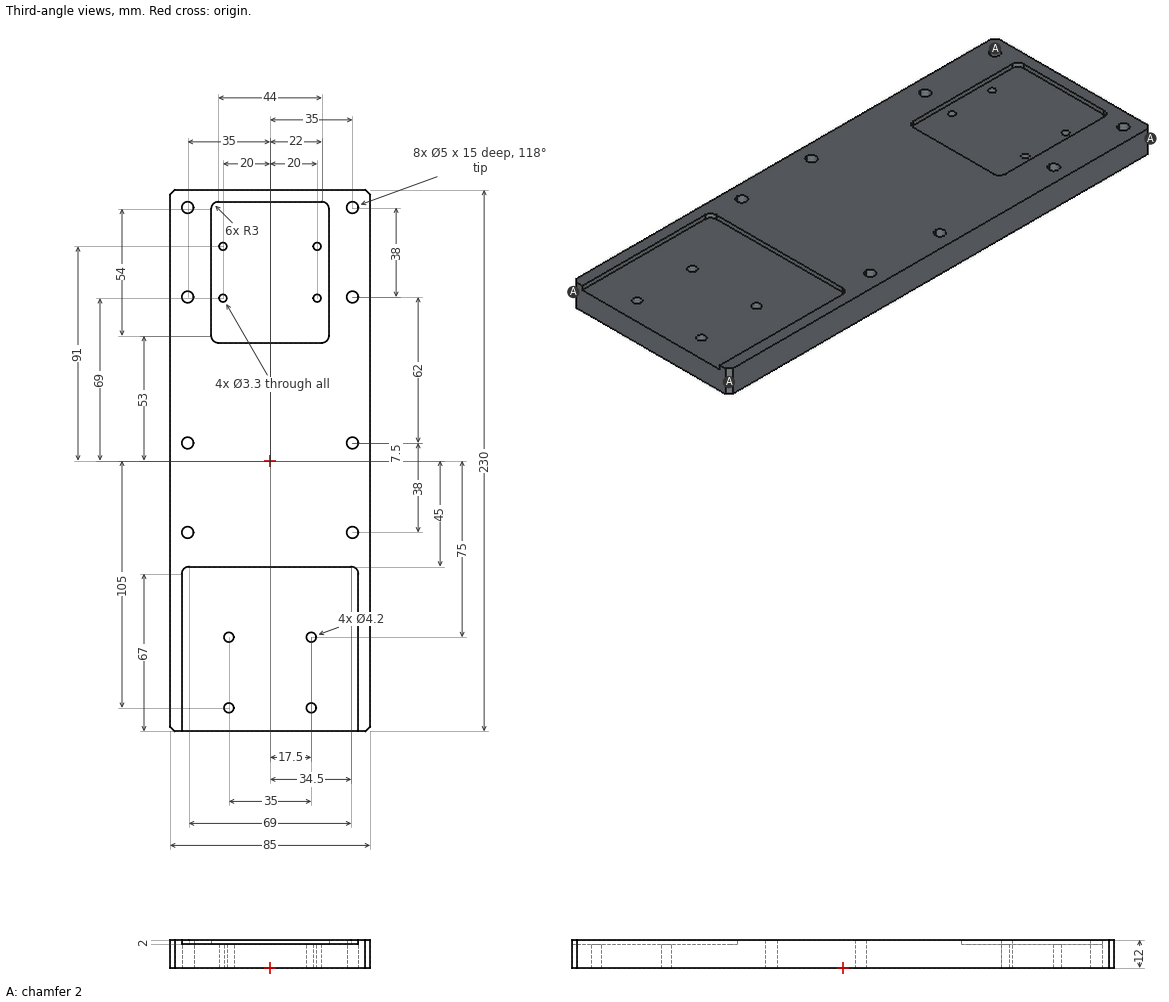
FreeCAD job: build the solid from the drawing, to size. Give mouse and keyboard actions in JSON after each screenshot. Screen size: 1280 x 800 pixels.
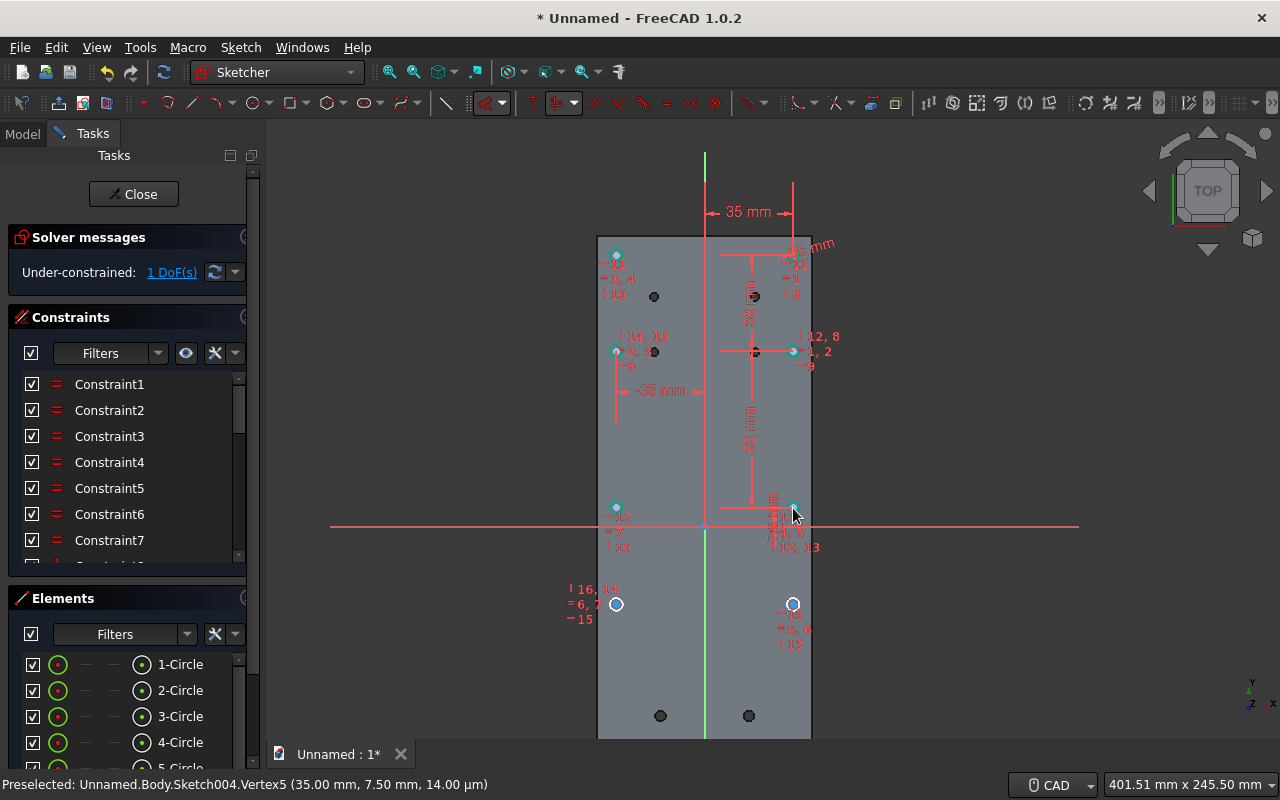
{"action": "left_click", "coordinate": [793, 508]}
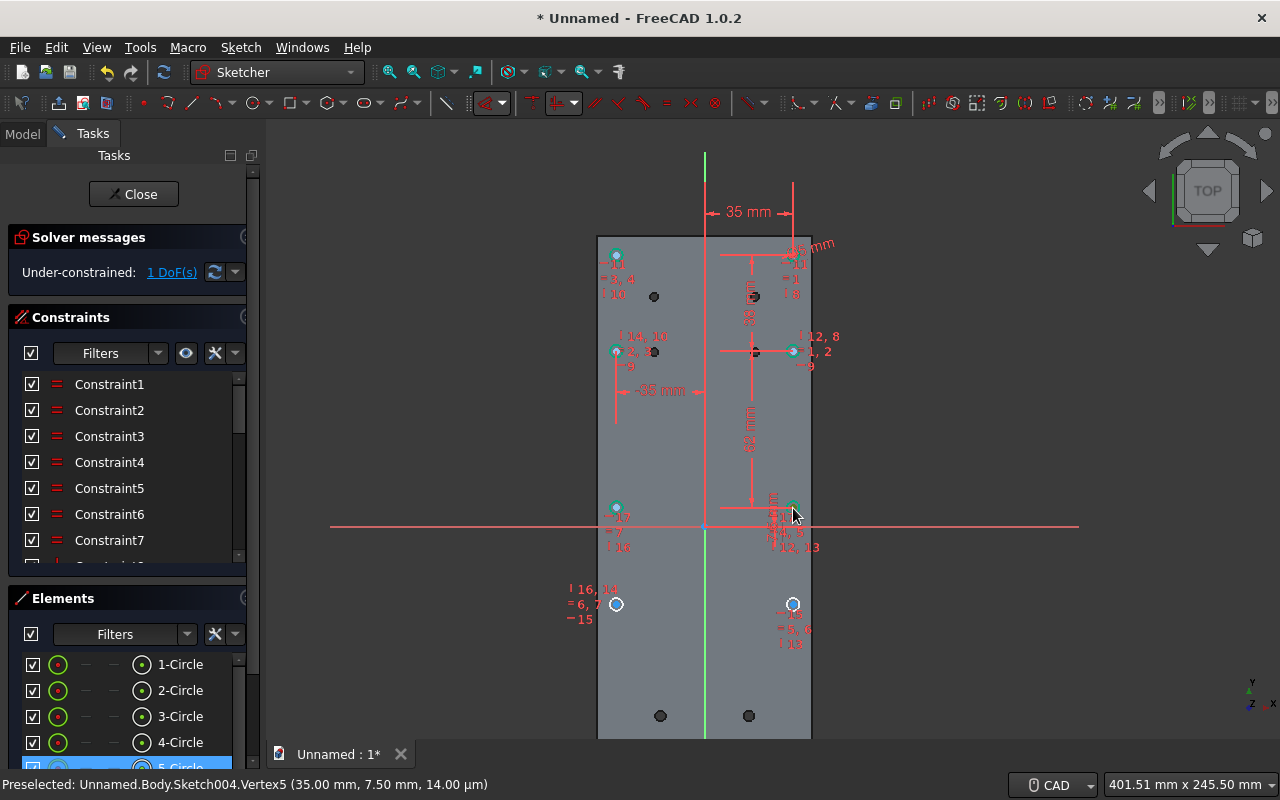
{"action": "left_click", "coordinate": [793, 604]}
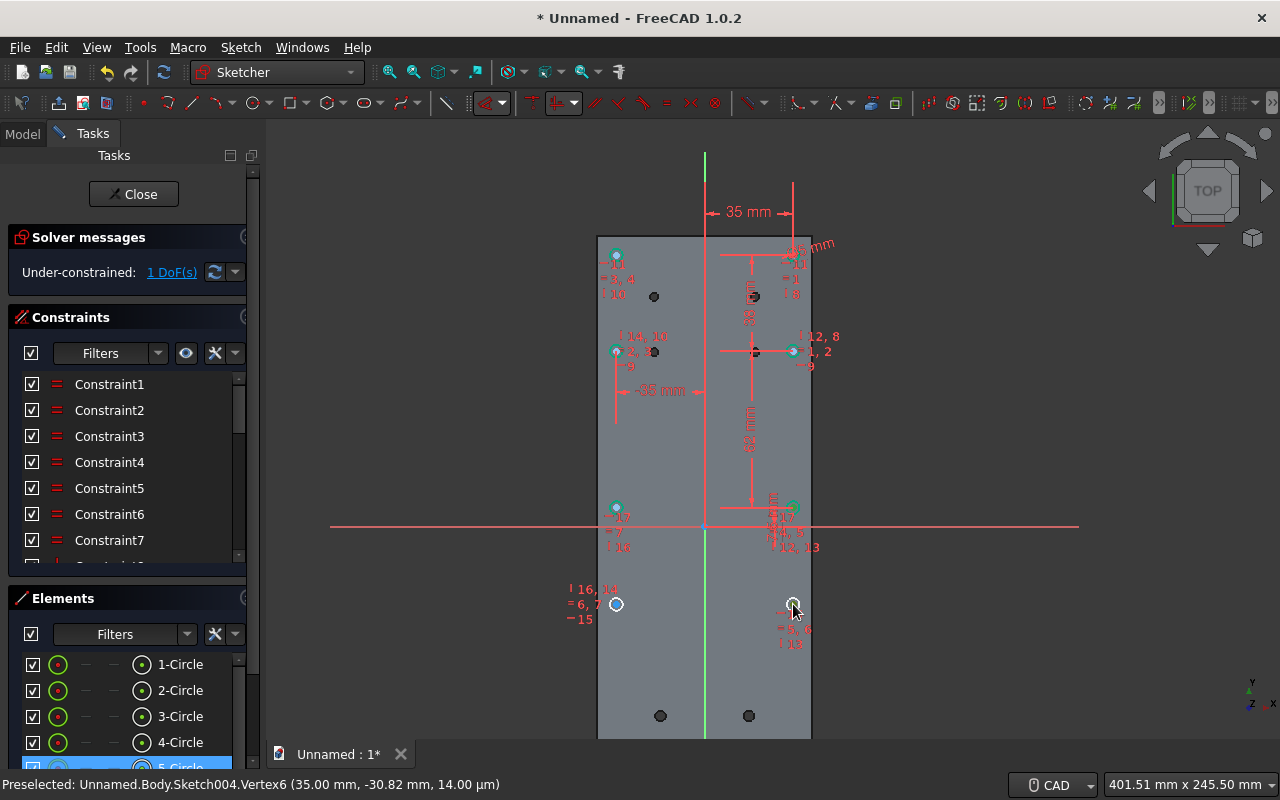
{"action": "key", "text": "i"}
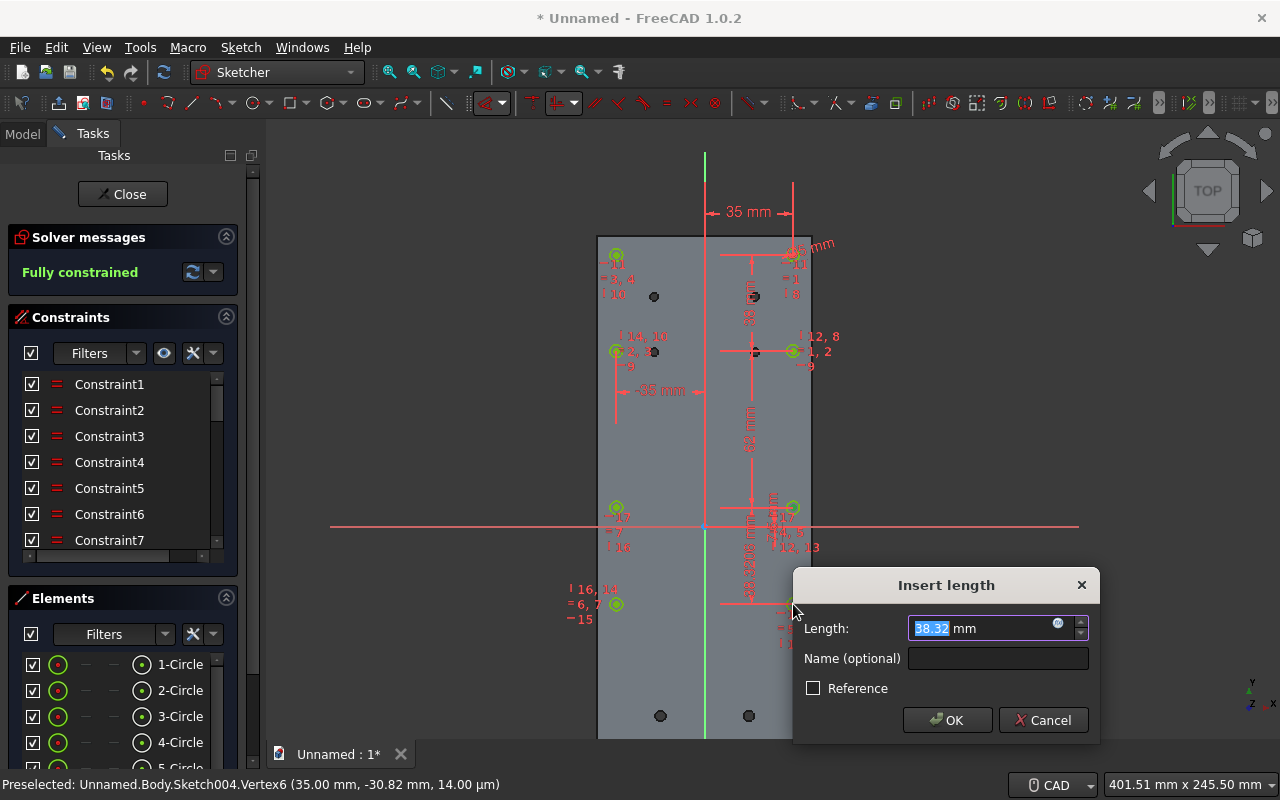
{"action": "type", "text": "38"}
{"action": "key", "text": "Return"}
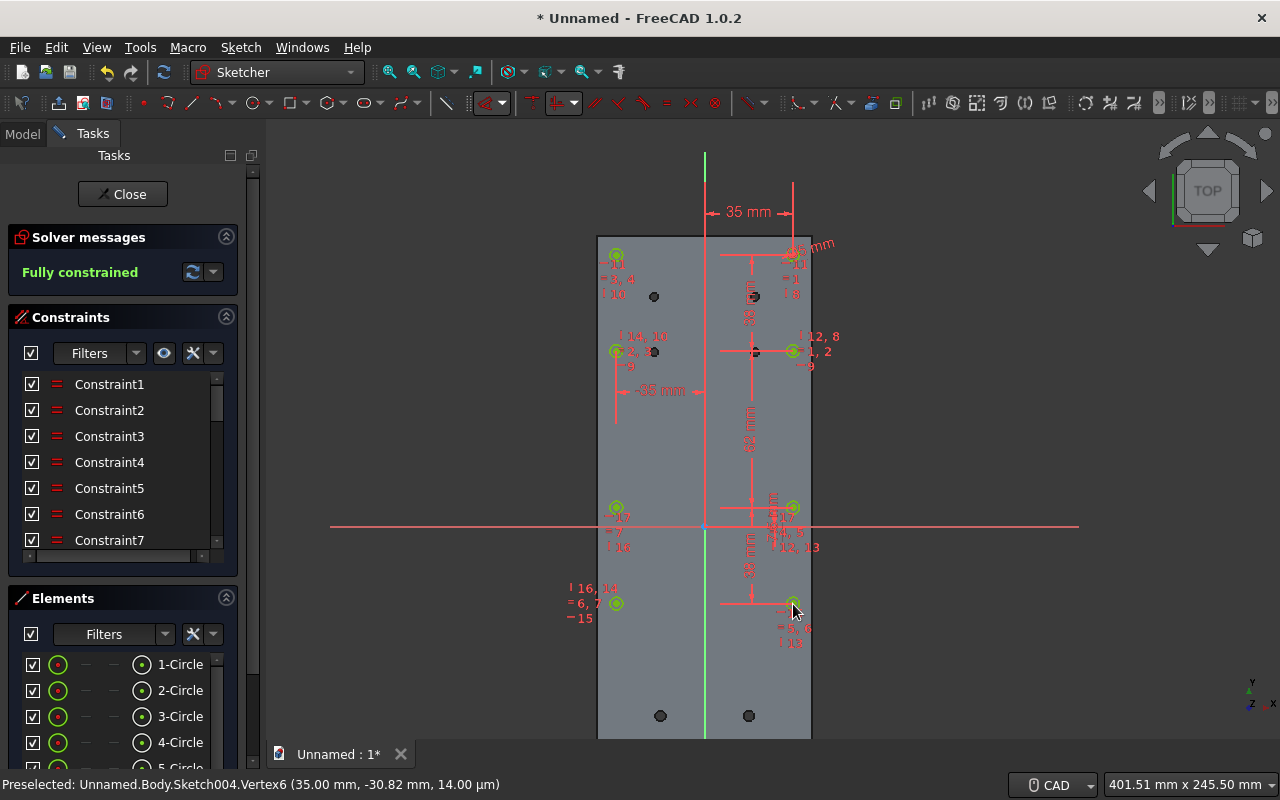
{"action": "left_click", "coordinate": [123, 194]}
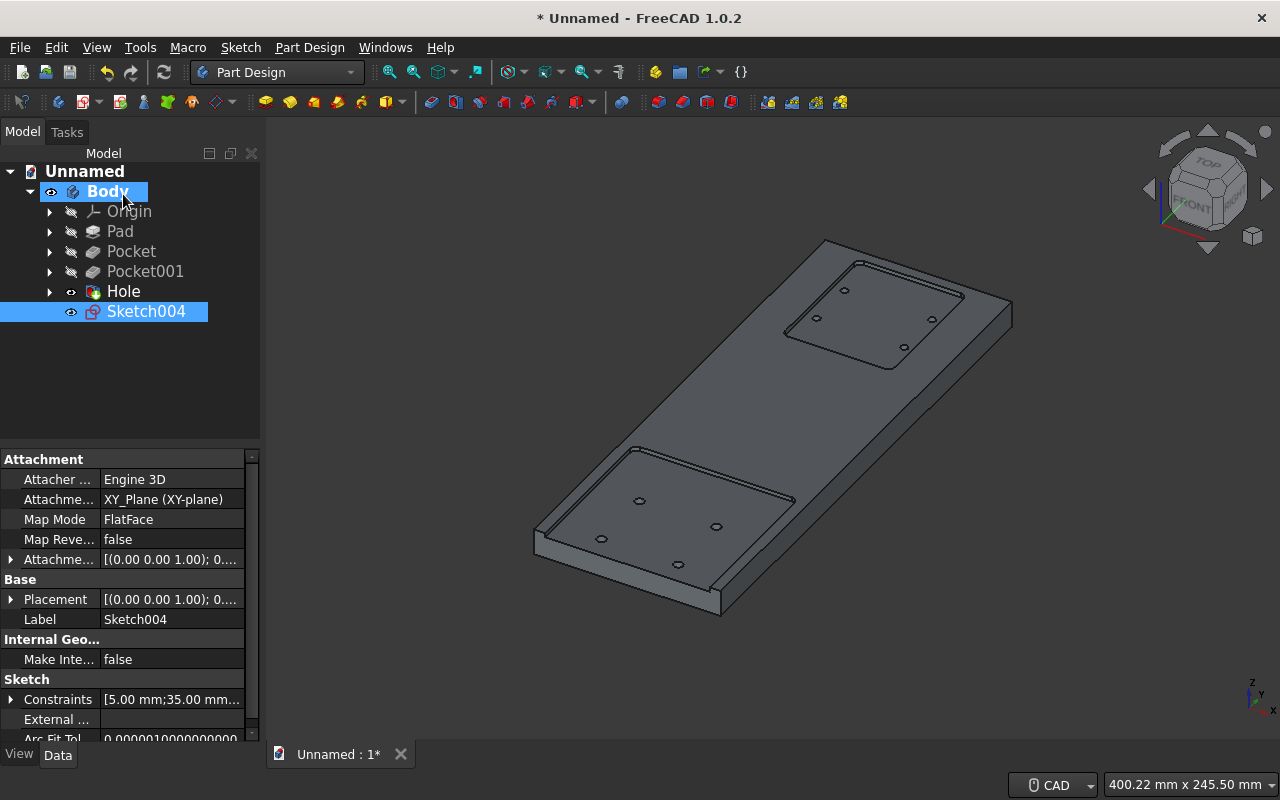
{"action": "left_click", "coordinate": [456, 102]}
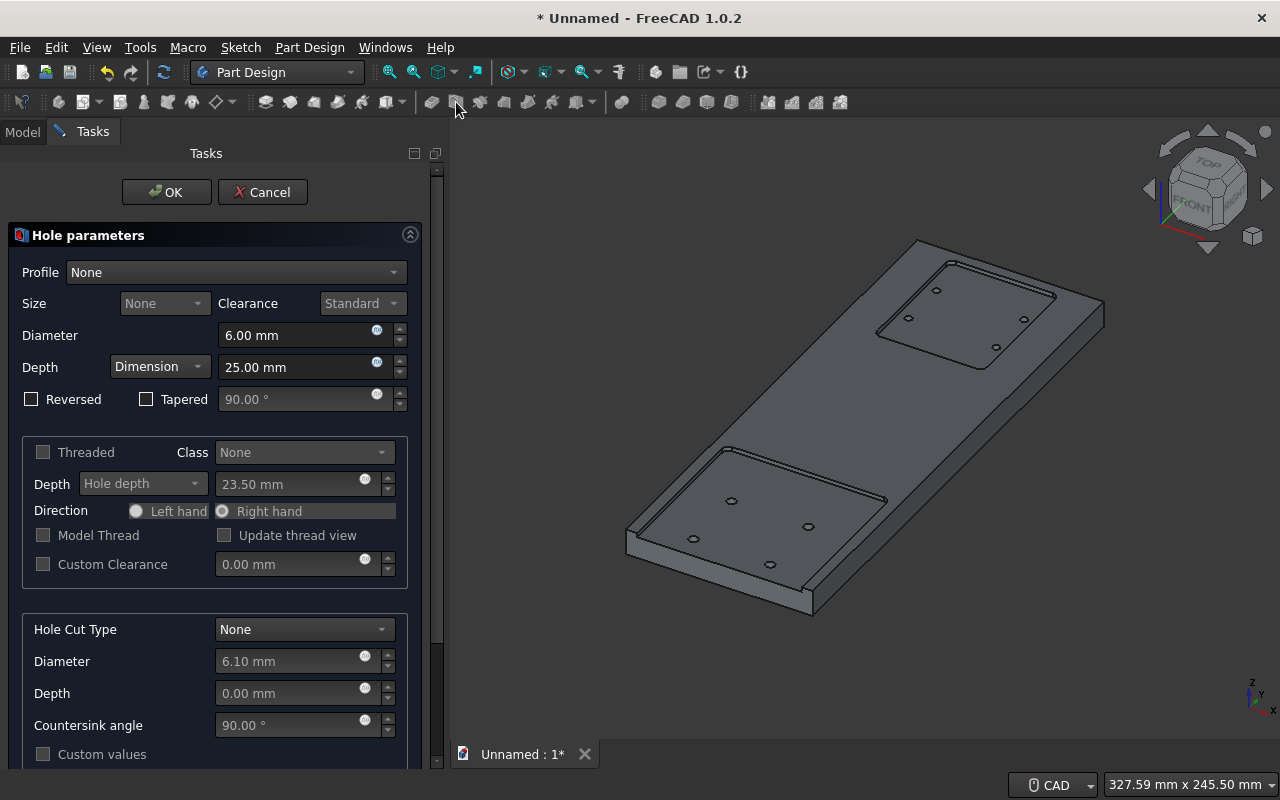
{"action": "triple_click", "coordinate": [305, 335]}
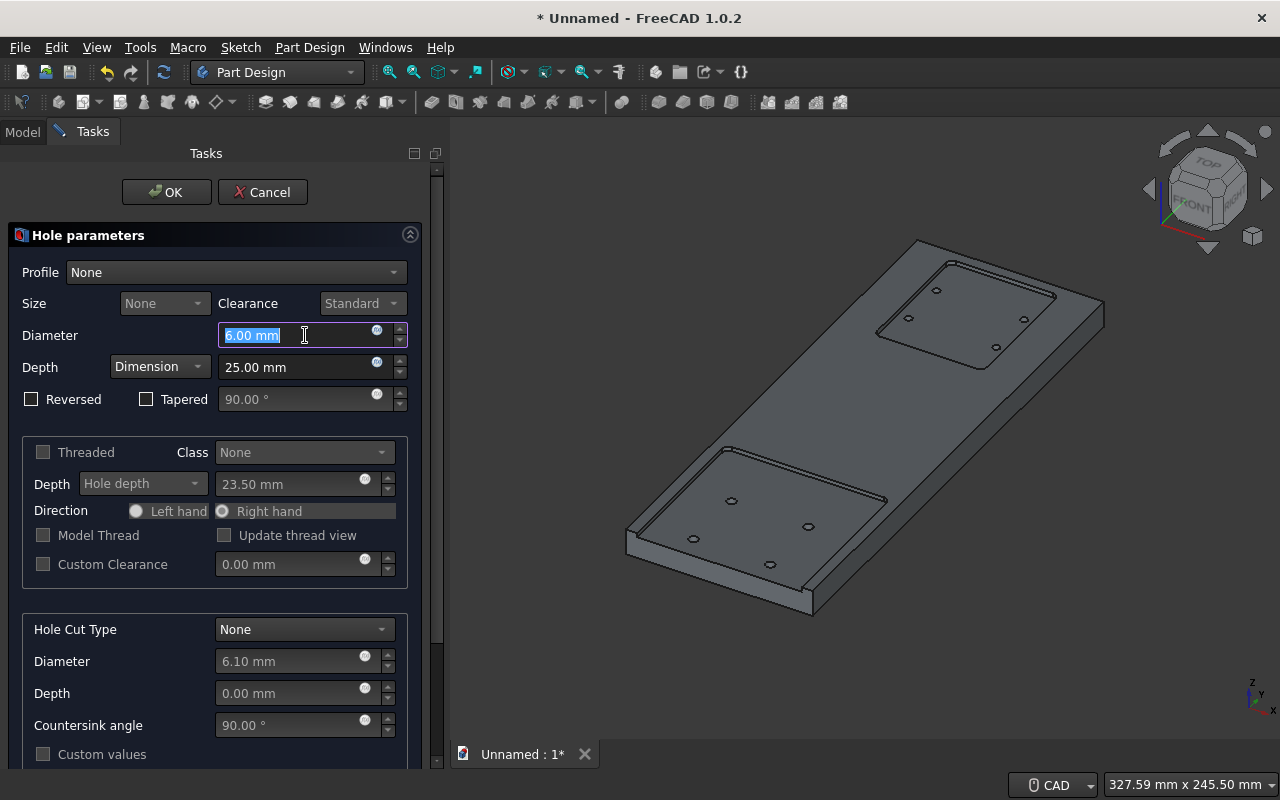
{"action": "type", "text": "5"}
{"action": "key", "text": "Tab"}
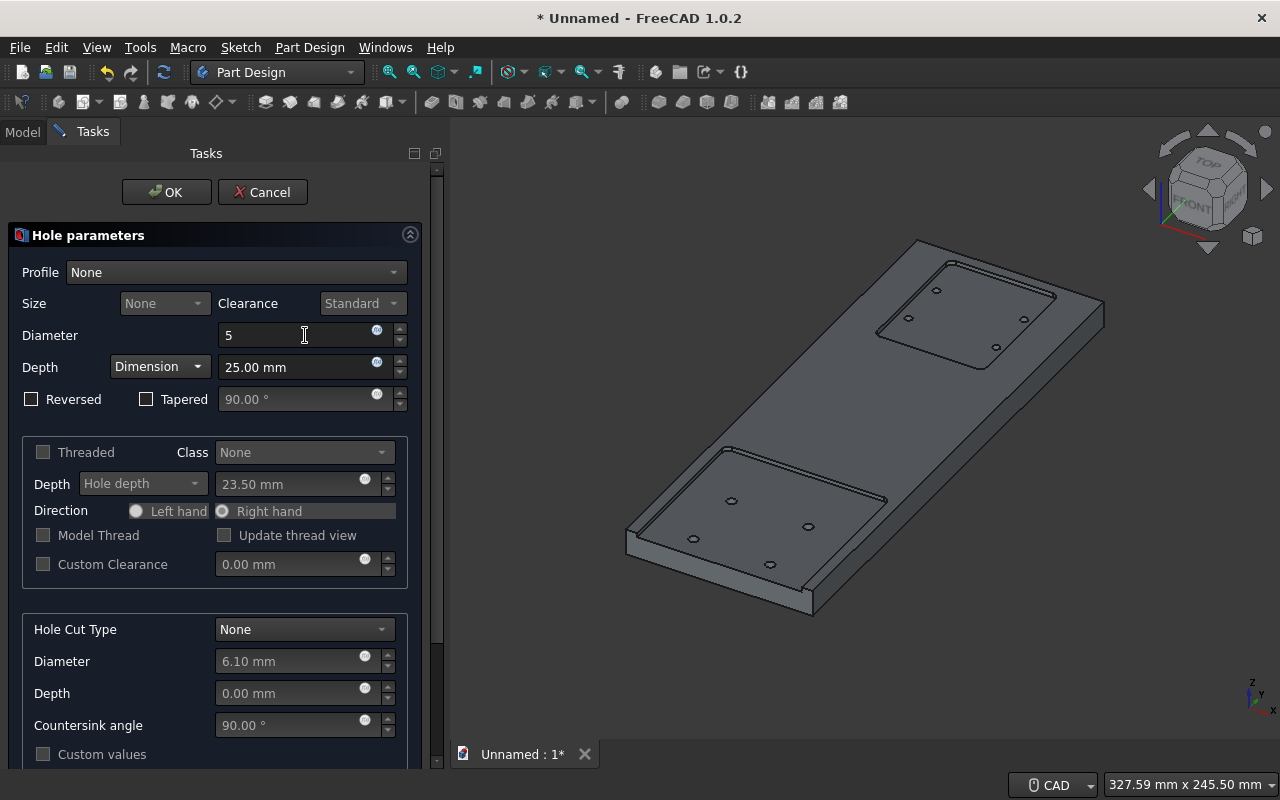
{"action": "triple_click", "coordinate": [305, 367]}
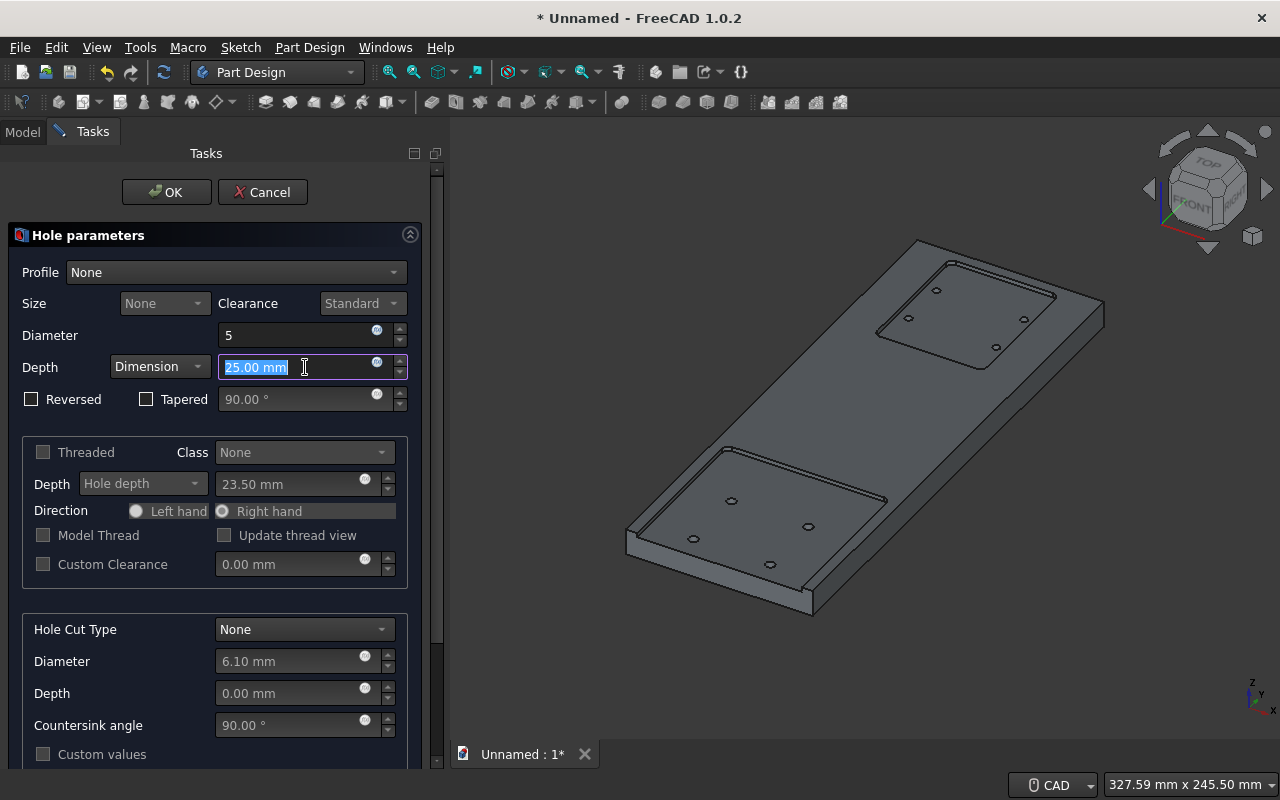
{"action": "type", "text": "15"}
{"action": "key", "text": "Tab"}